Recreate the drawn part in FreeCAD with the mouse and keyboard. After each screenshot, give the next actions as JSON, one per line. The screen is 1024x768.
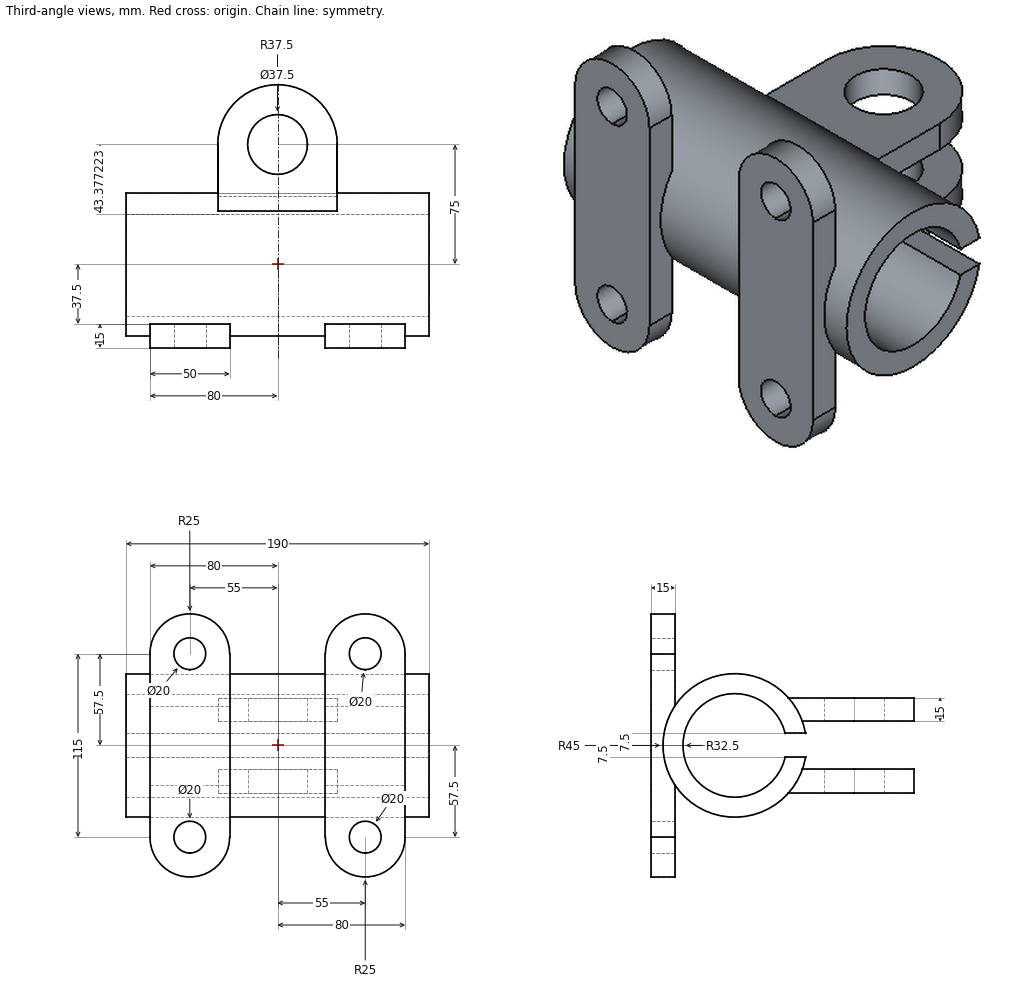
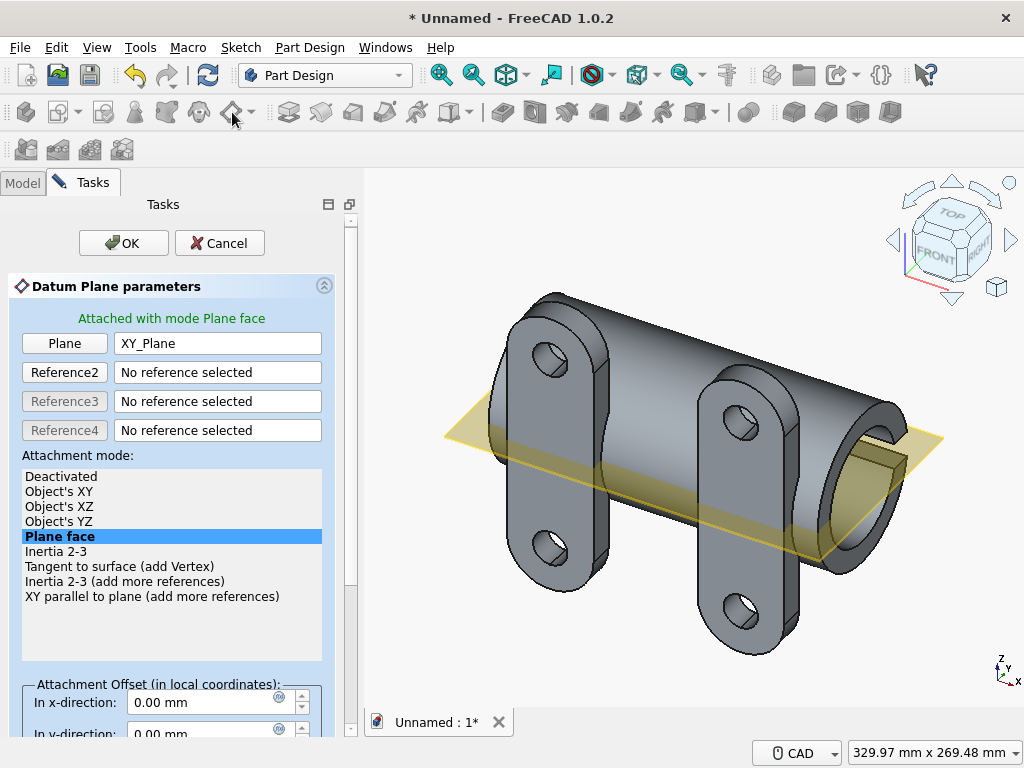
{"action": "scroll", "coordinate": [351, 475], "scroll_direction": "down", "scroll_amount": 2}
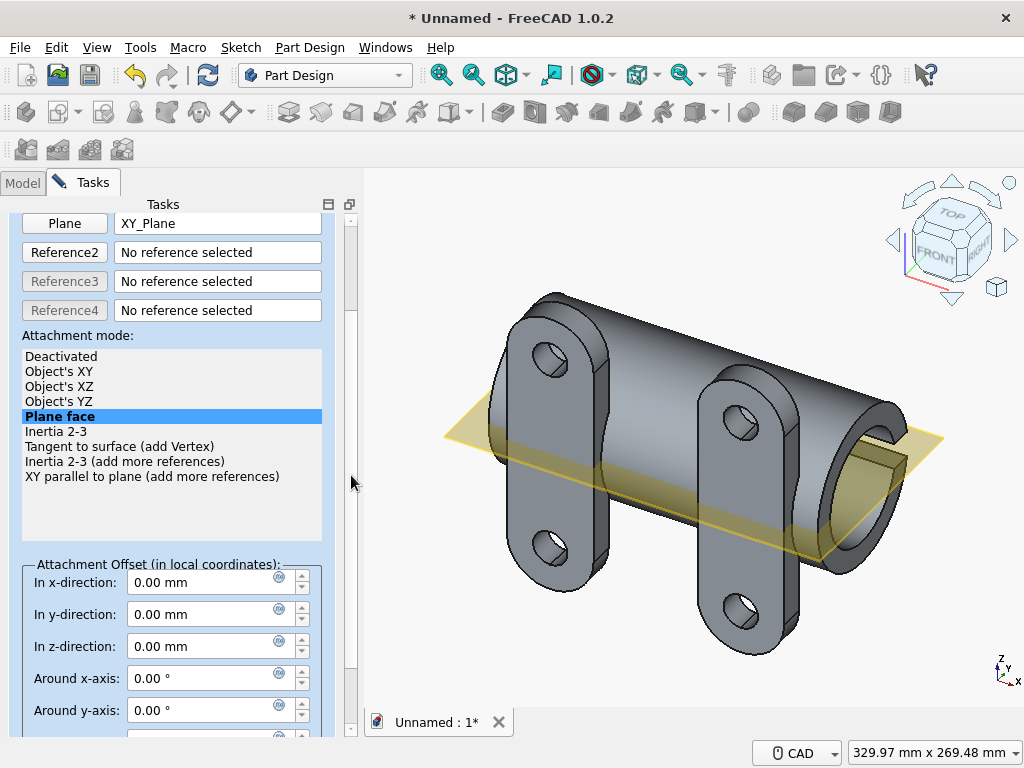
{"action": "triple_click", "coordinate": [210, 646]}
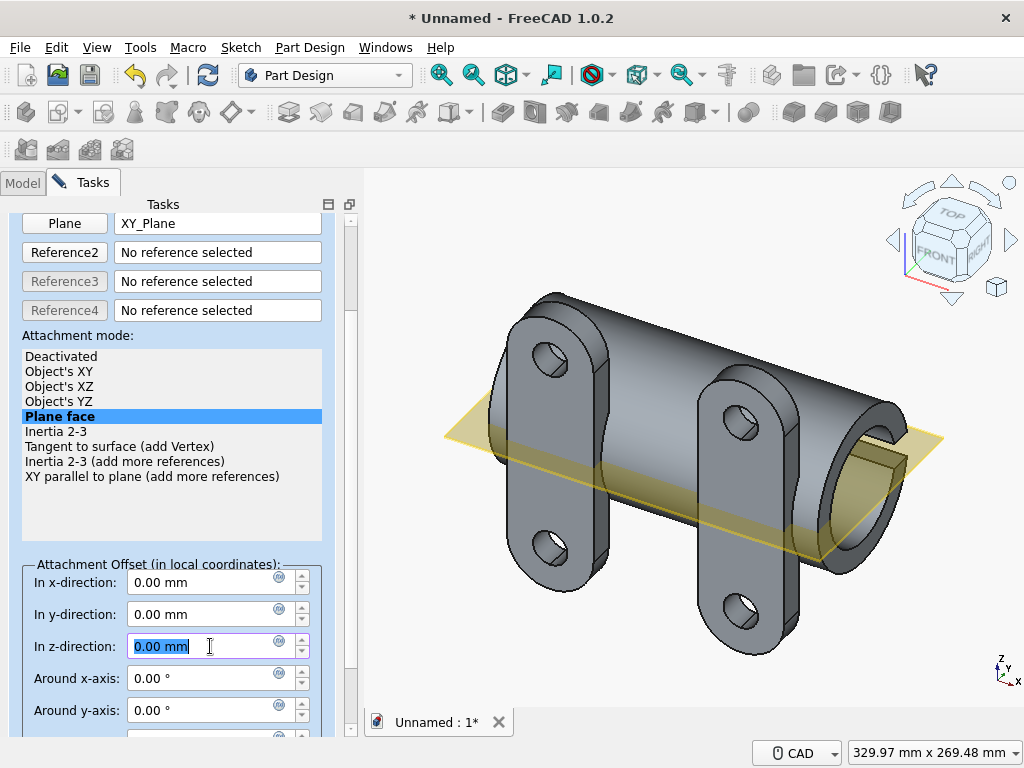
{"action": "type", "text": "15"}
{"action": "key", "text": "Tab"}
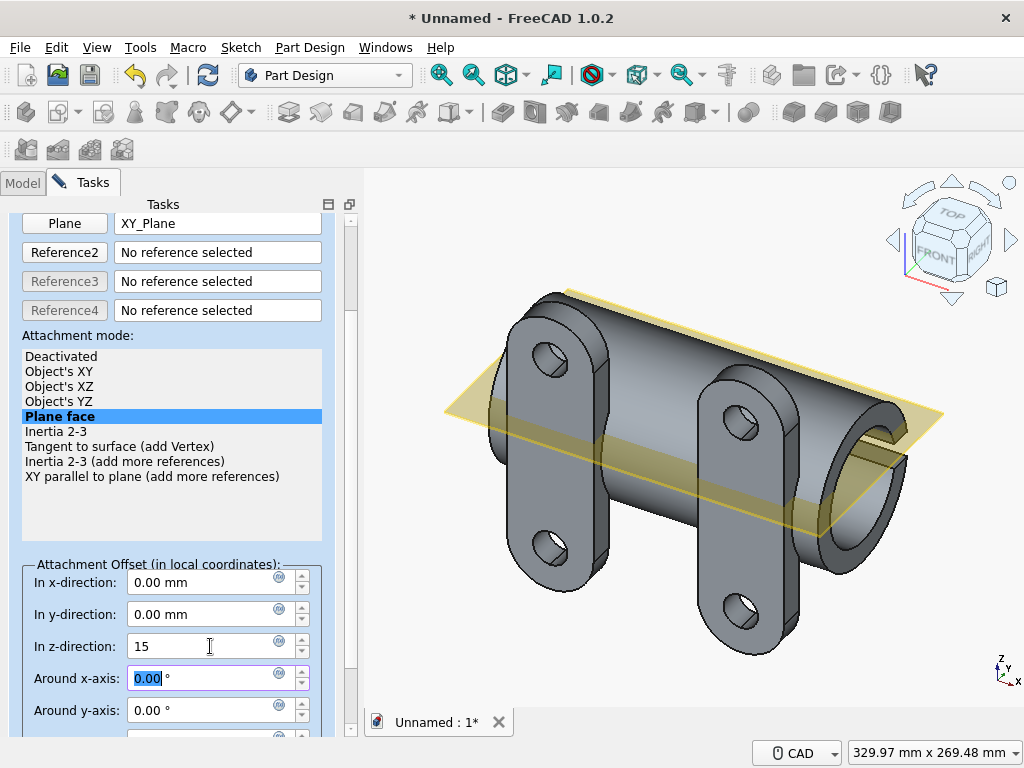
{"action": "scroll", "coordinate": [351, 475], "scroll_direction": "up", "scroll_amount": 3}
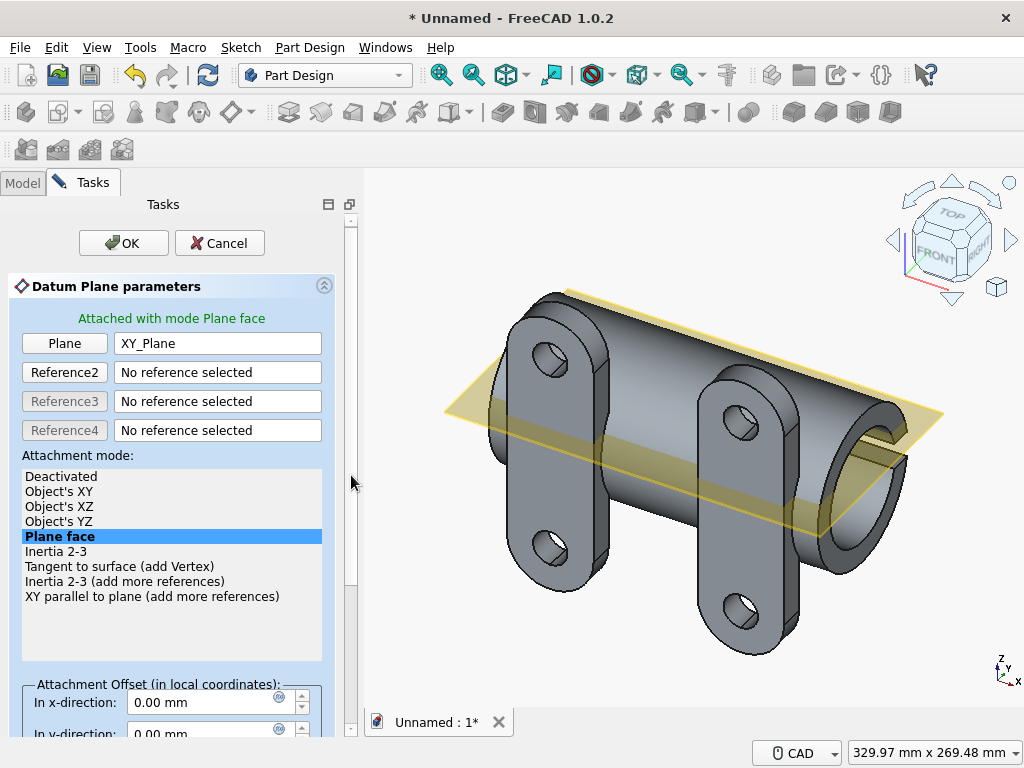
{"action": "left_click", "coordinate": [124, 243]}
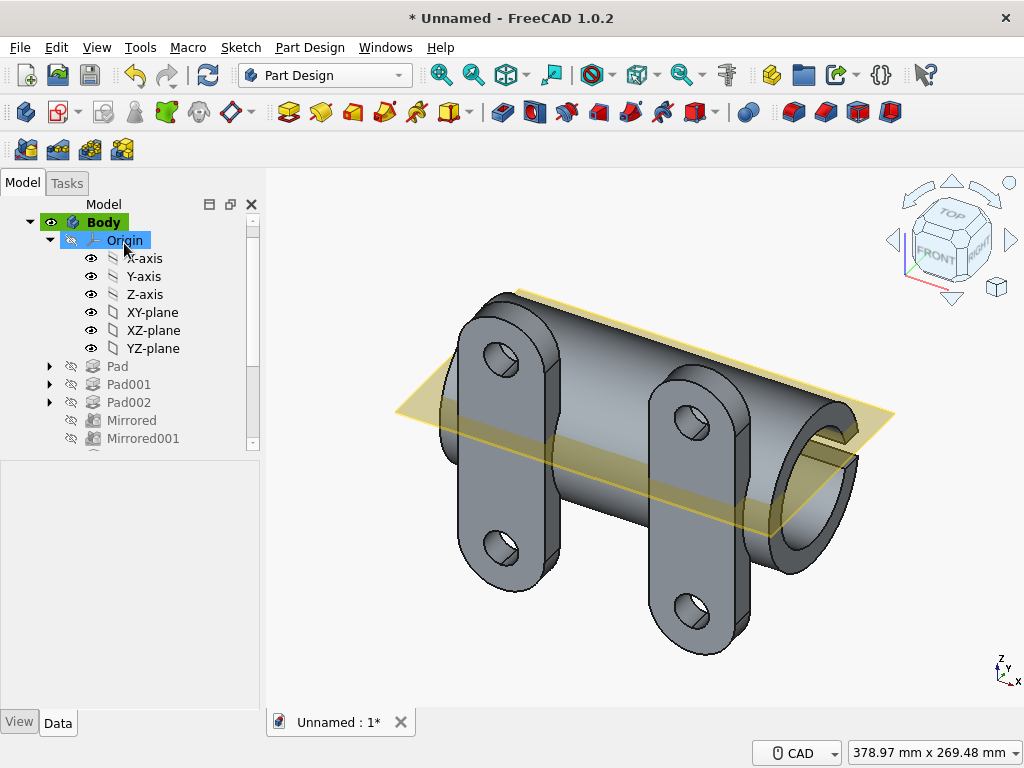
{"action": "scroll", "coordinate": [120, 326], "scroll_direction": "down", "scroll_amount": 3}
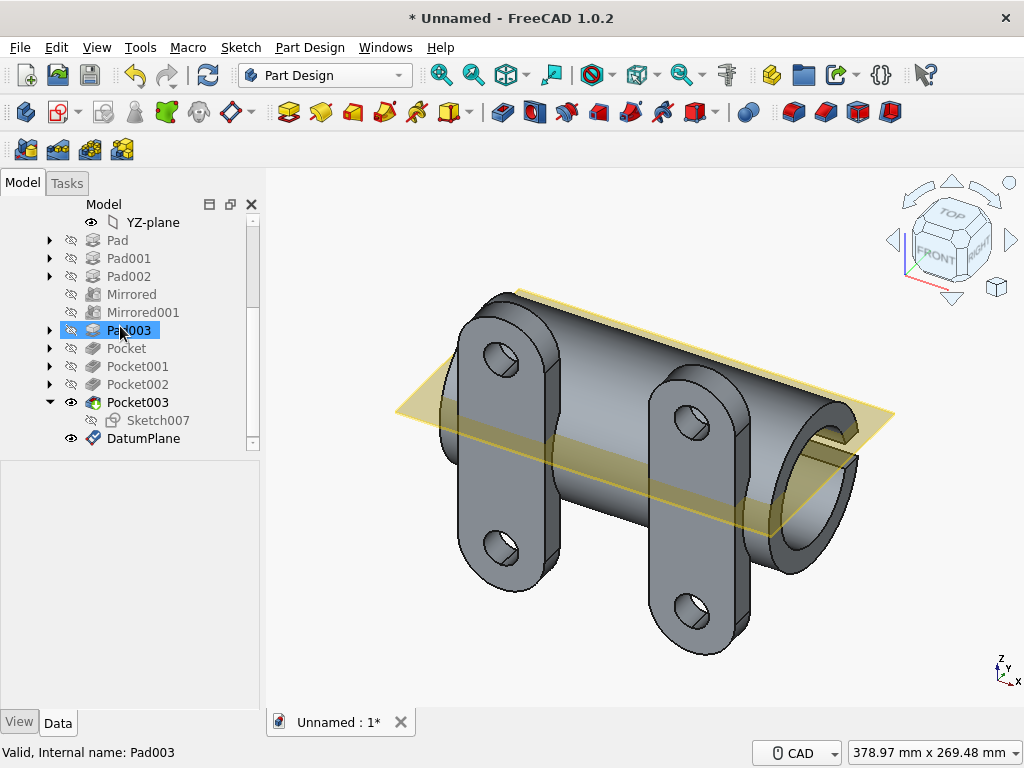
{"action": "left_click", "coordinate": [116, 438]}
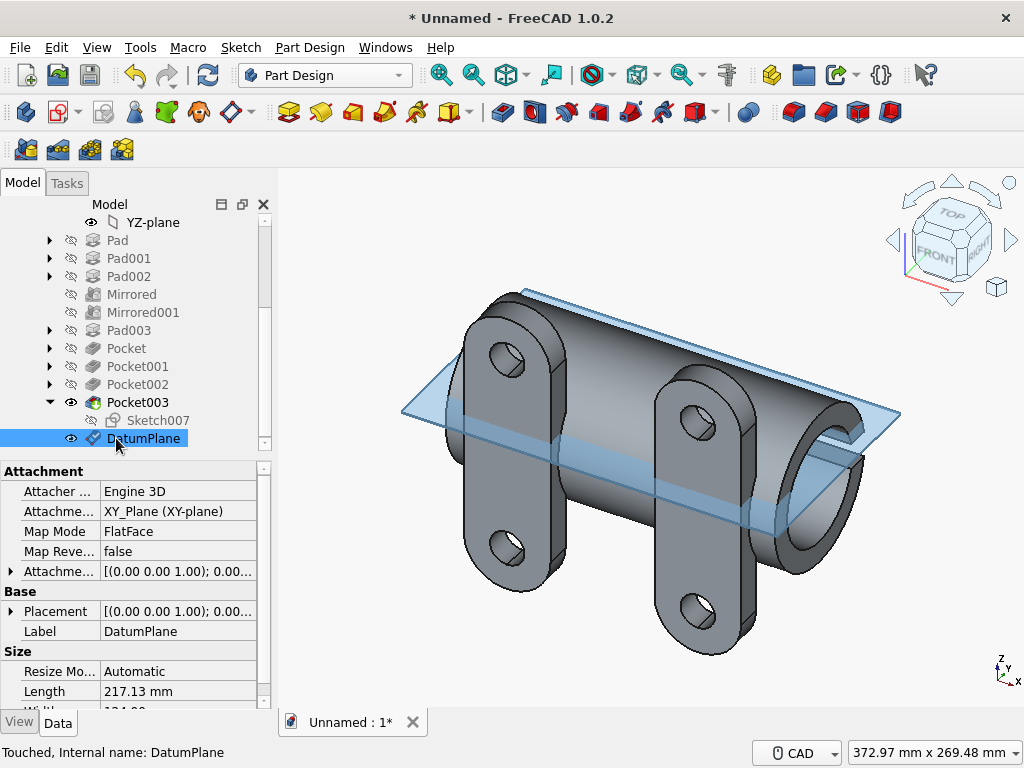
{"action": "left_click", "coordinate": [58, 112]}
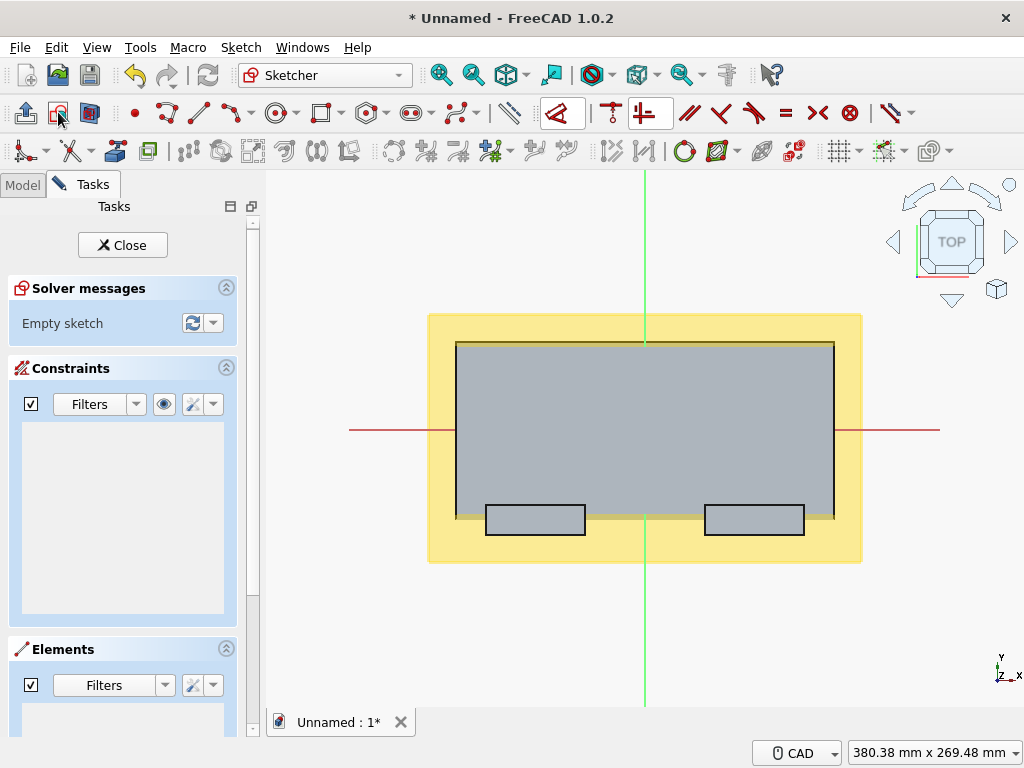
{"action": "left_click", "coordinate": [90, 114]}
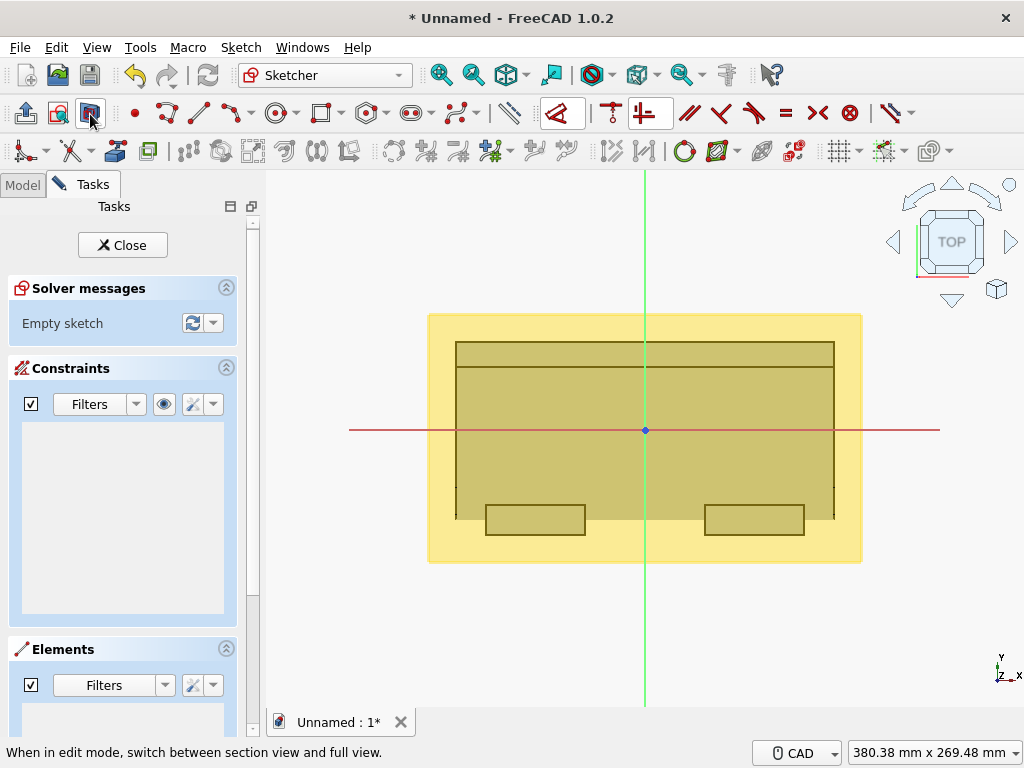
{"action": "scroll", "coordinate": [294, 679], "scroll_direction": "down", "scroll_amount": 1}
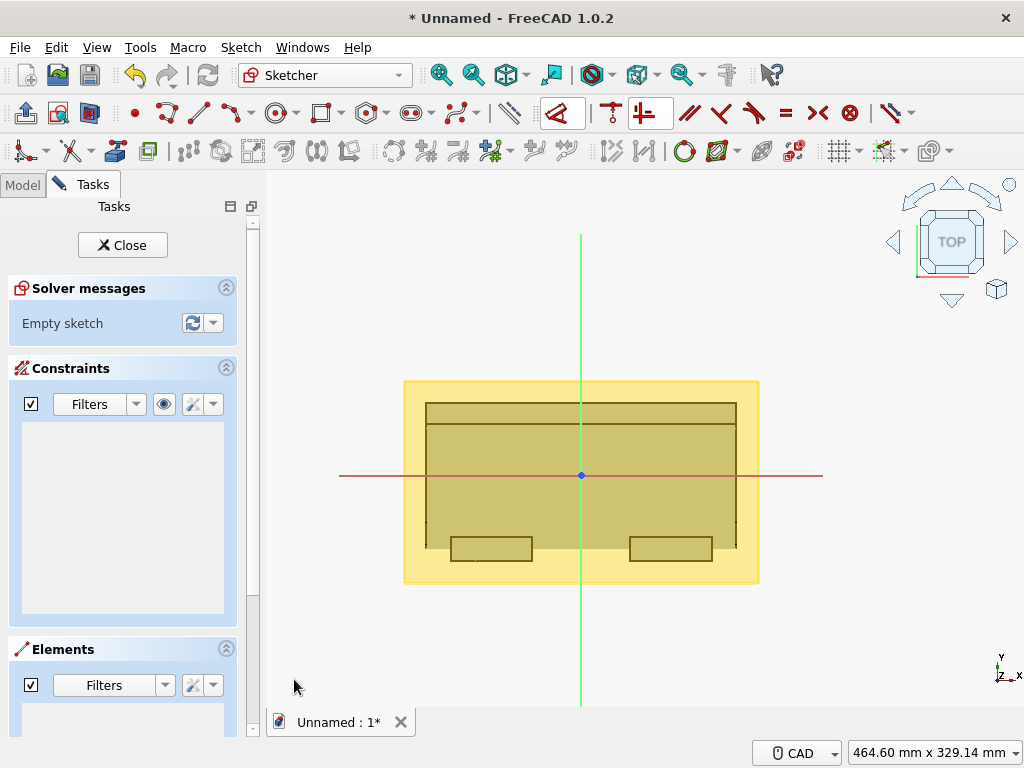
{"action": "scroll", "coordinate": [587, 317], "scroll_direction": "up", "scroll_amount": 3}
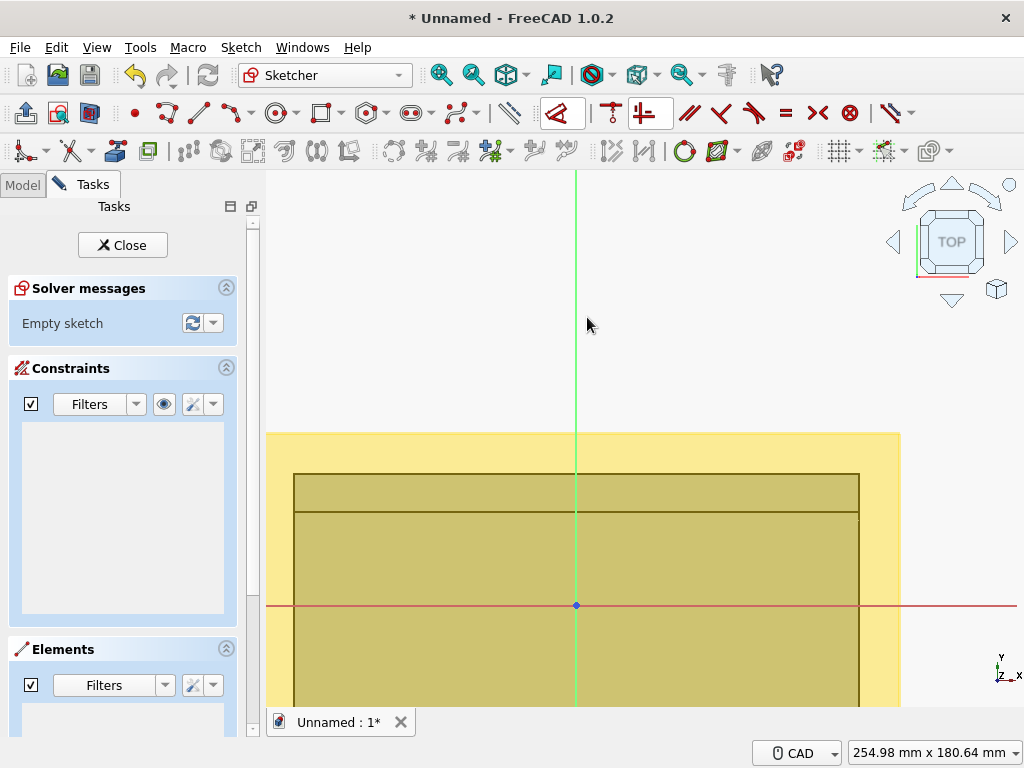
{"action": "left_click", "coordinate": [168, 114]}